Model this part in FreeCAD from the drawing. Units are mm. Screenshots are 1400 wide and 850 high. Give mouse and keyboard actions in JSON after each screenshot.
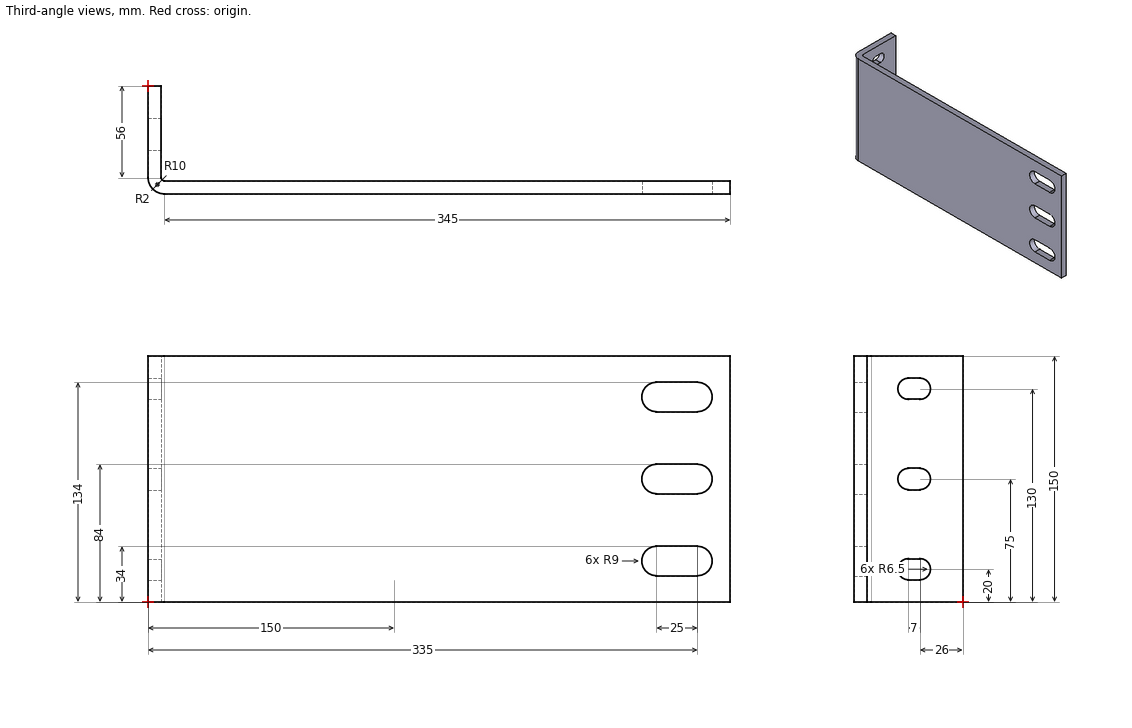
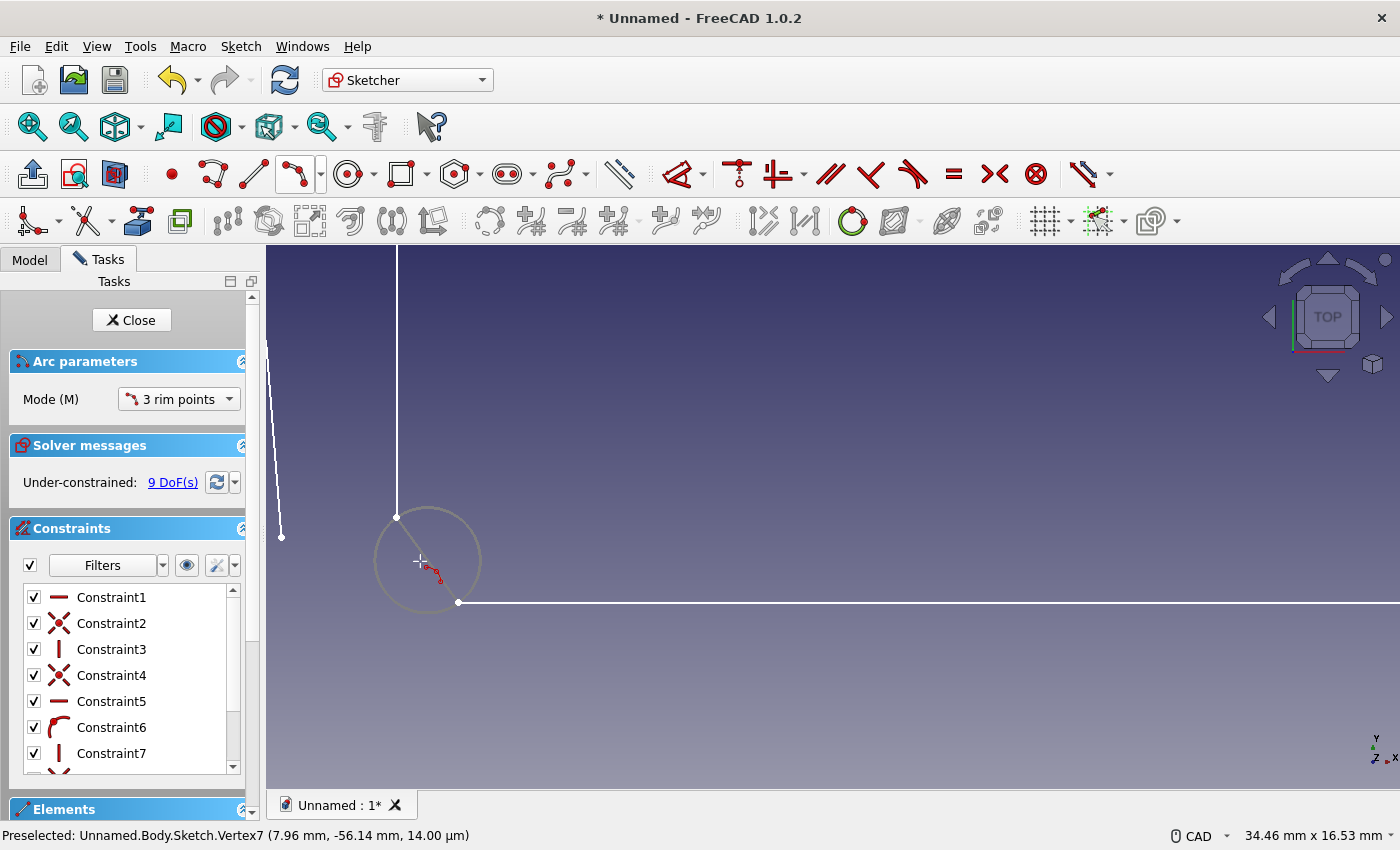
{"action": "left_click", "coordinate": [417, 560]}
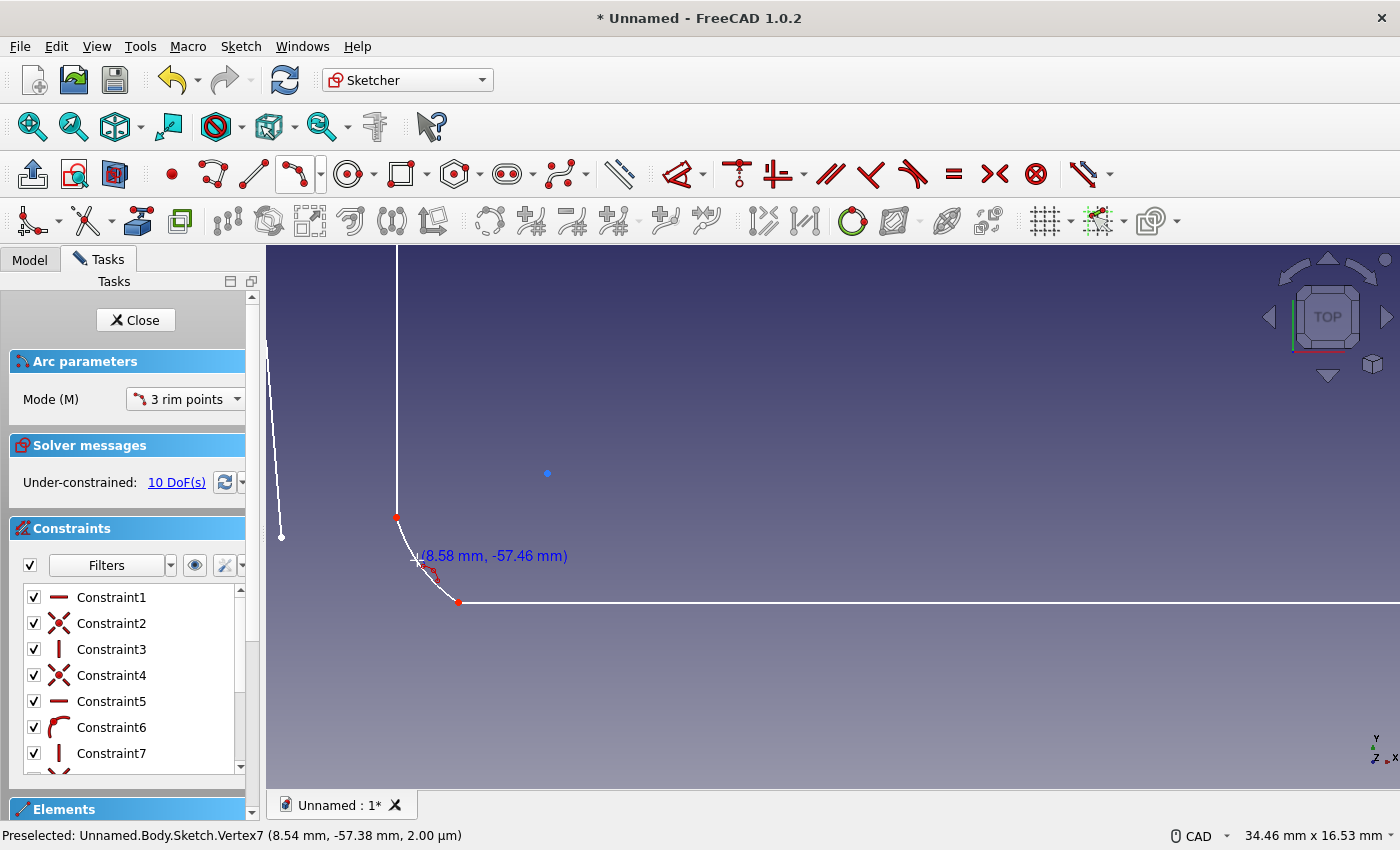
{"action": "scroll", "coordinate": [427, 566], "scroll_direction": "down", "scroll_amount": 14}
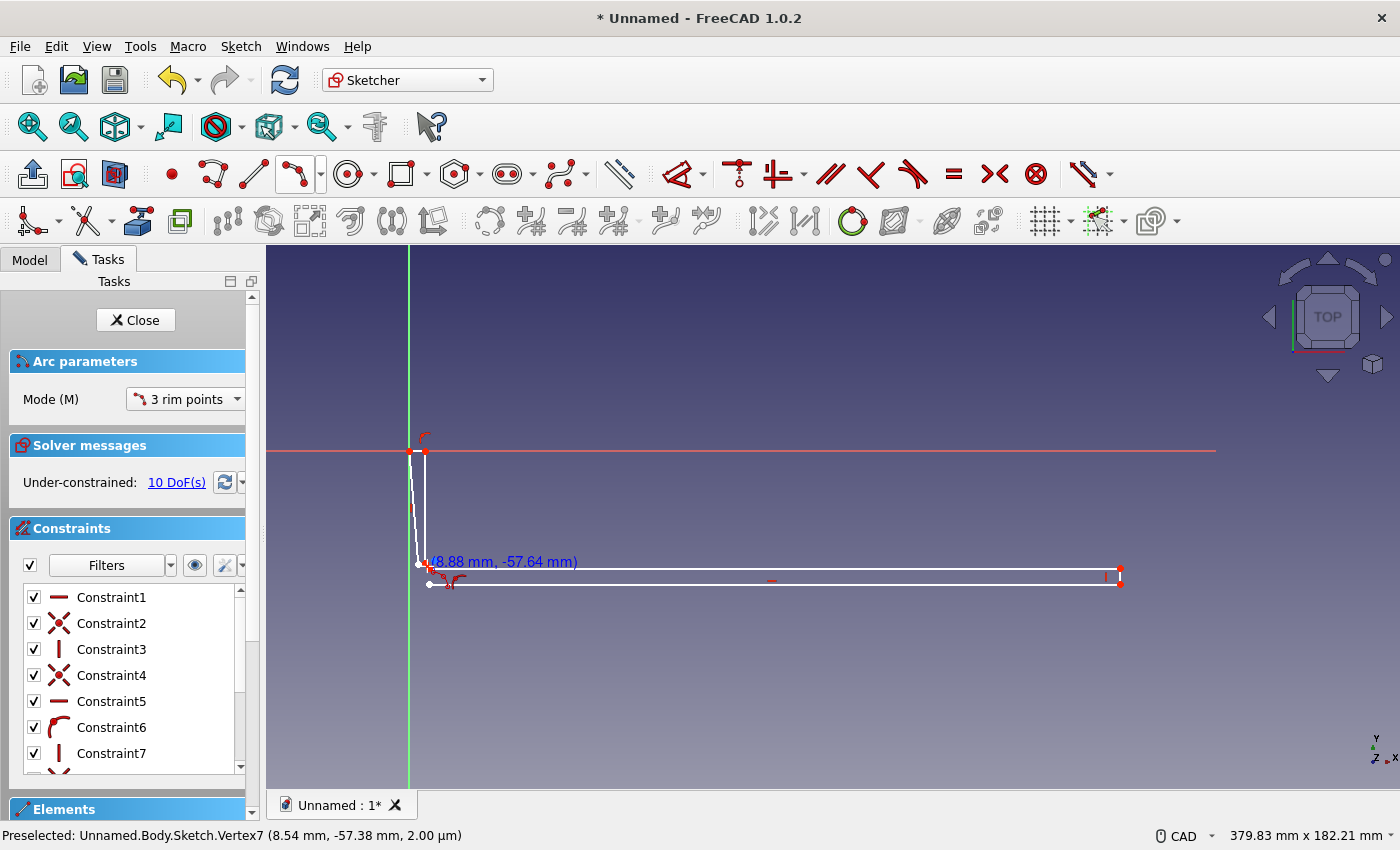
{"action": "left_click", "coordinate": [418, 565]}
{"action": "left_click", "coordinate": [429, 585]}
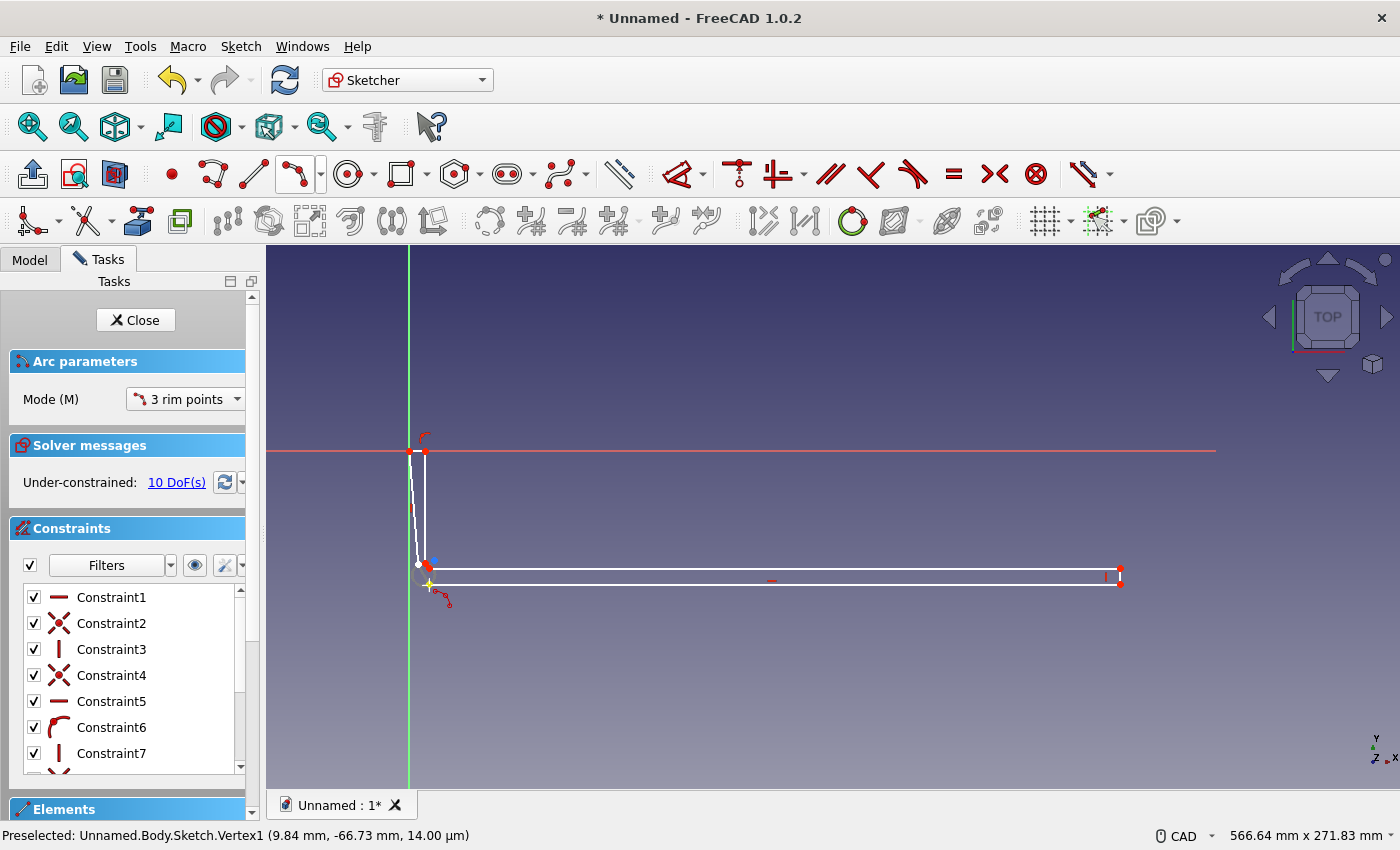
{"action": "scroll", "coordinate": [415, 577], "scroll_direction": "up", "scroll_amount": 5}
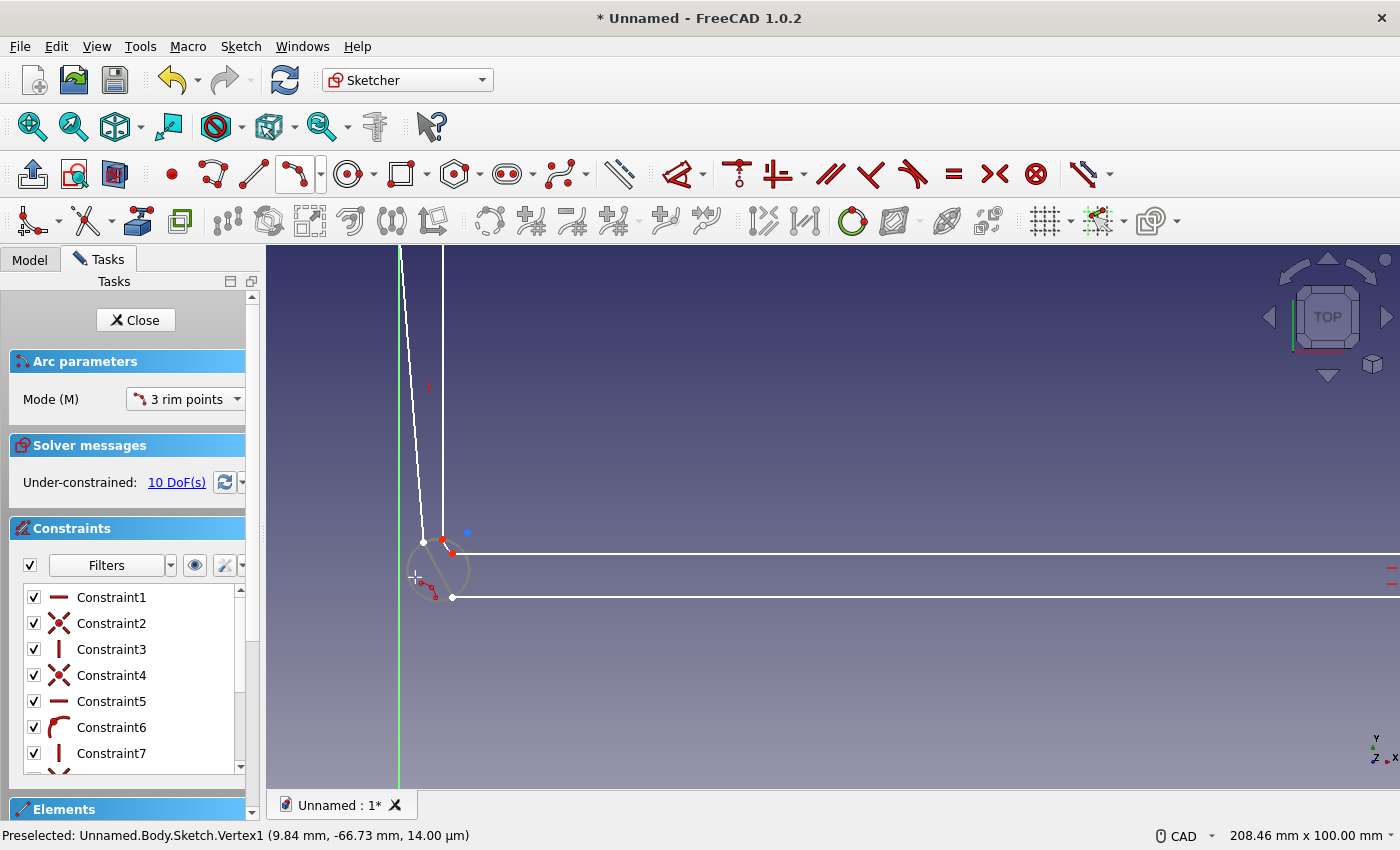
{"action": "left_click", "coordinate": [415, 577]}
{"action": "key", "text": "Escape"}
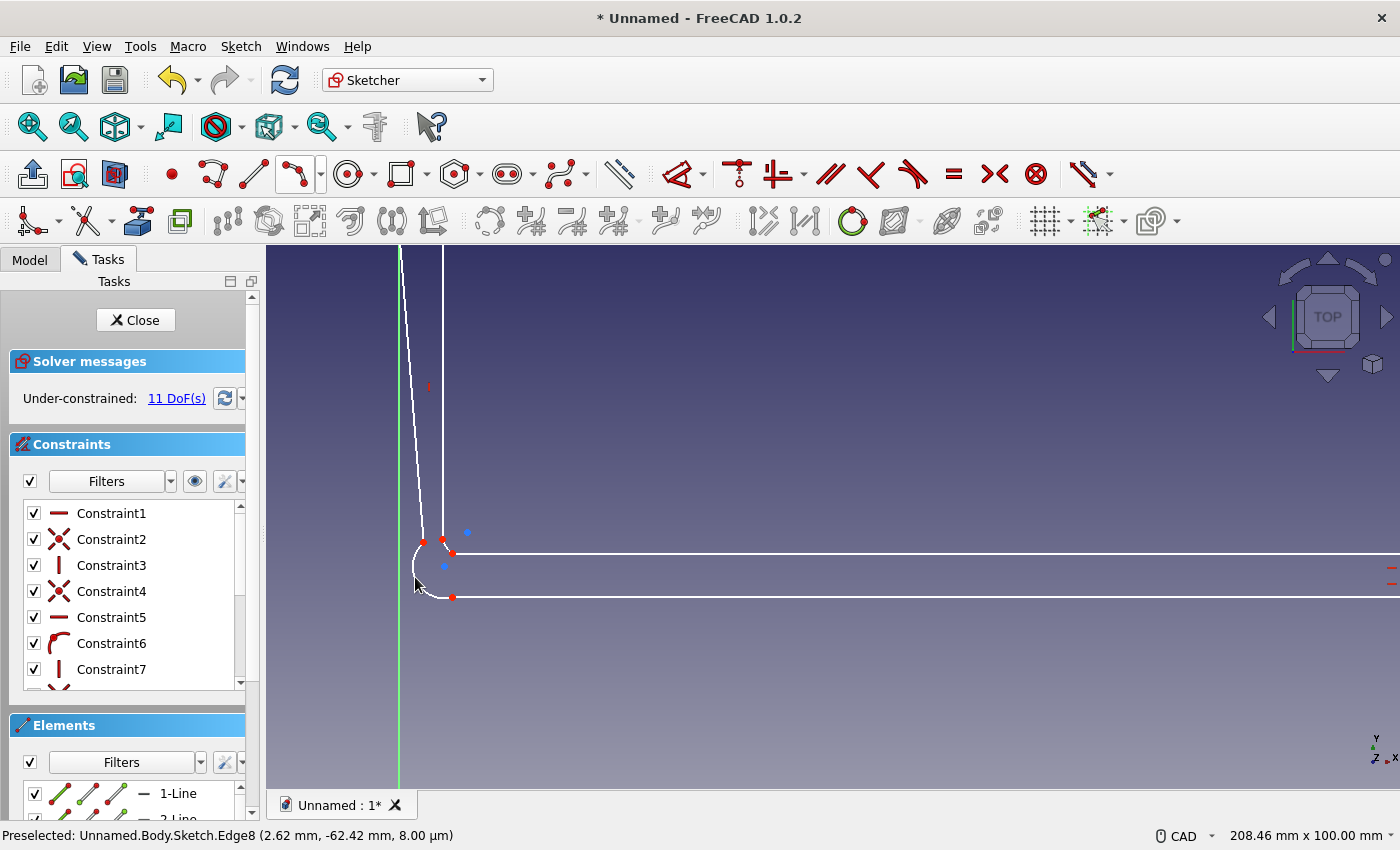
{"action": "left_click", "coordinate": [1016, 597]}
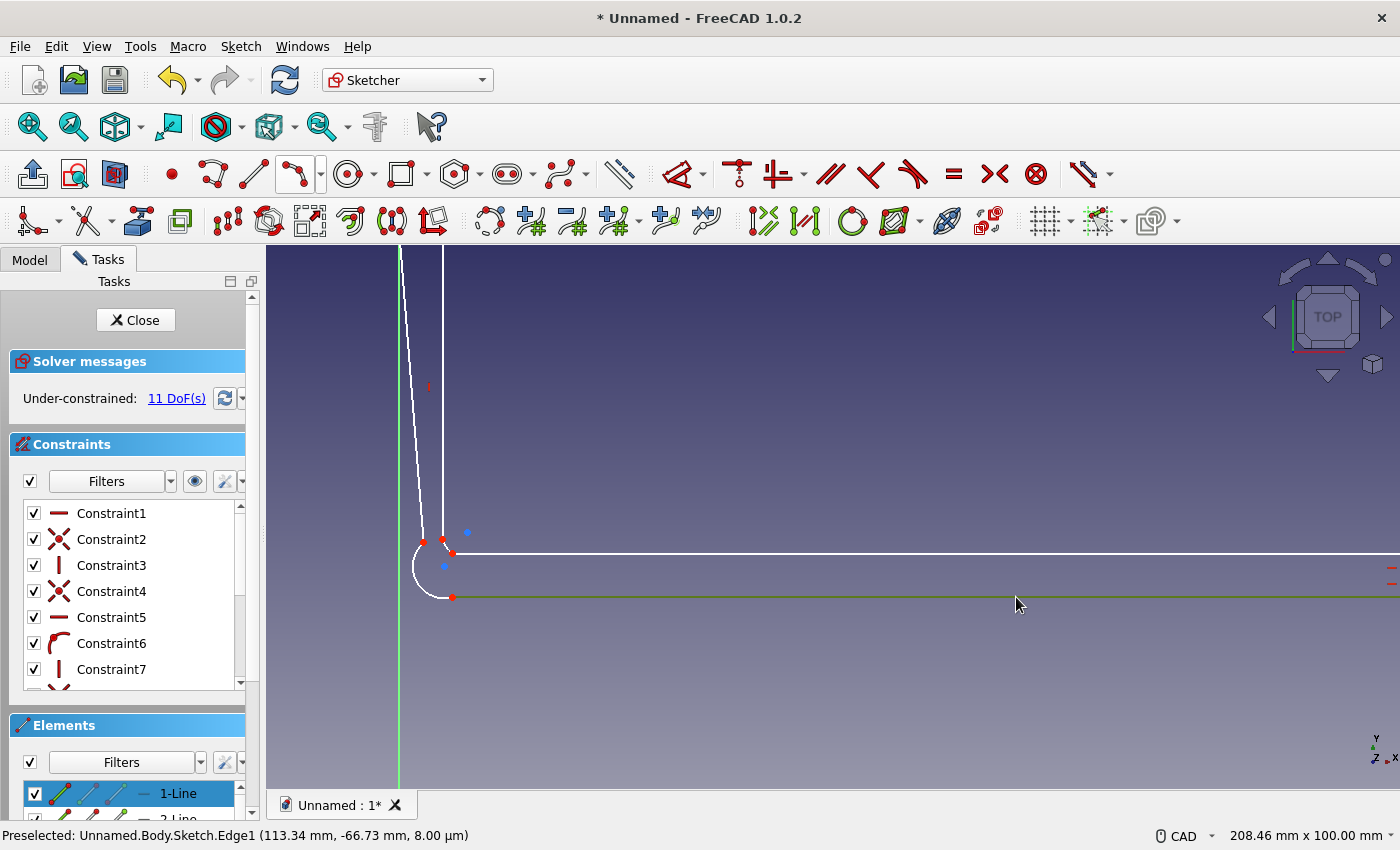
{"action": "left_click", "coordinate": [413, 565]}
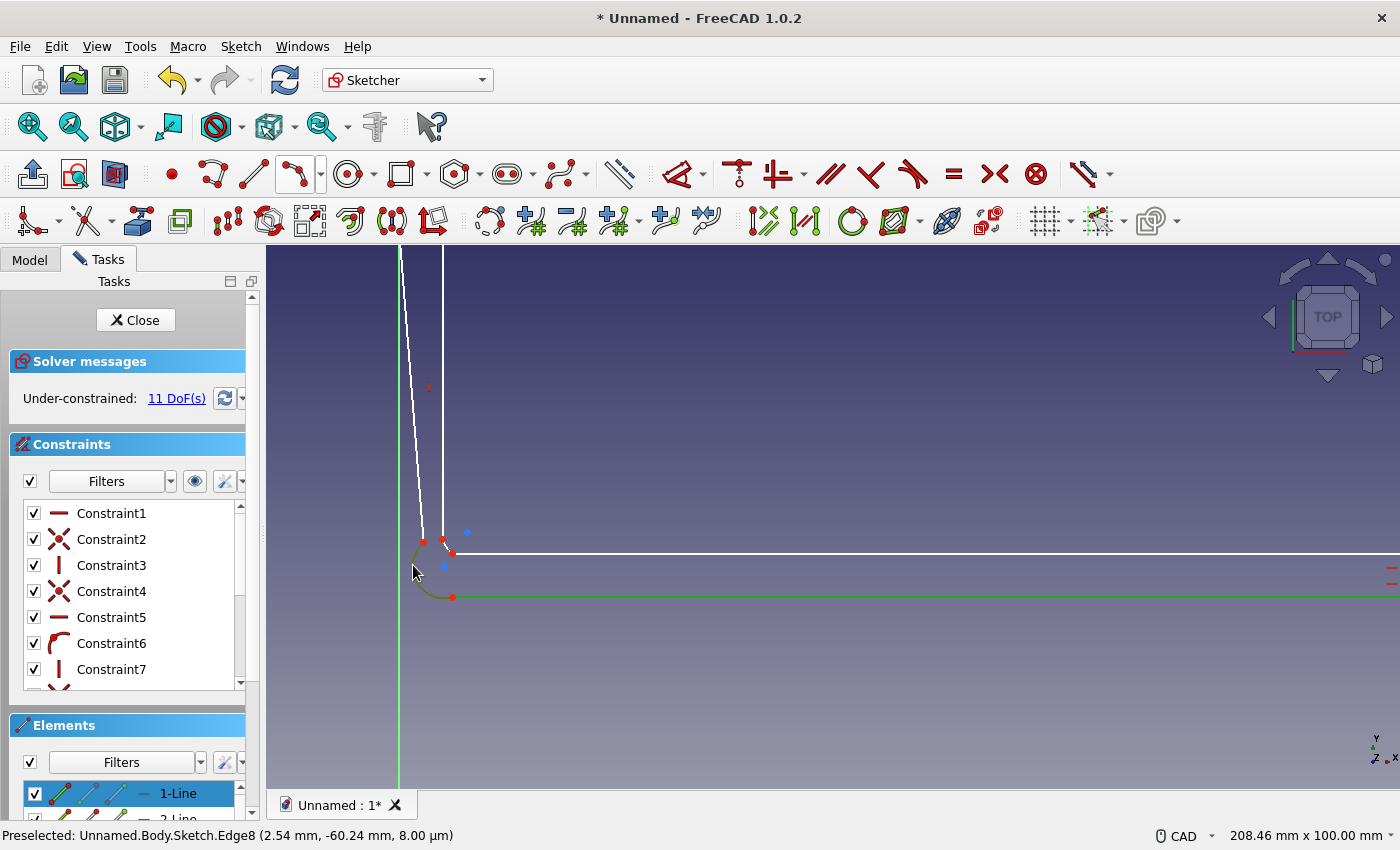
{"action": "left_click", "coordinate": [913, 174]}